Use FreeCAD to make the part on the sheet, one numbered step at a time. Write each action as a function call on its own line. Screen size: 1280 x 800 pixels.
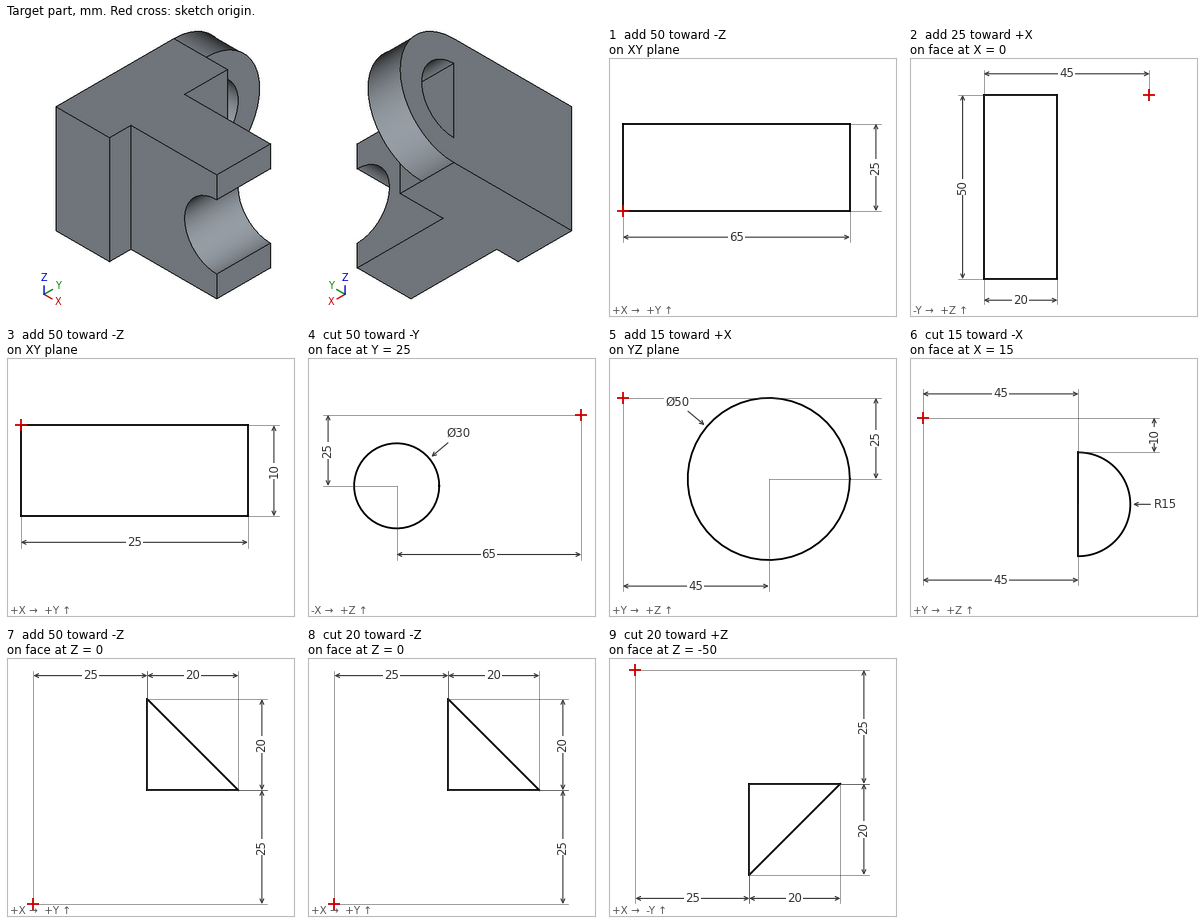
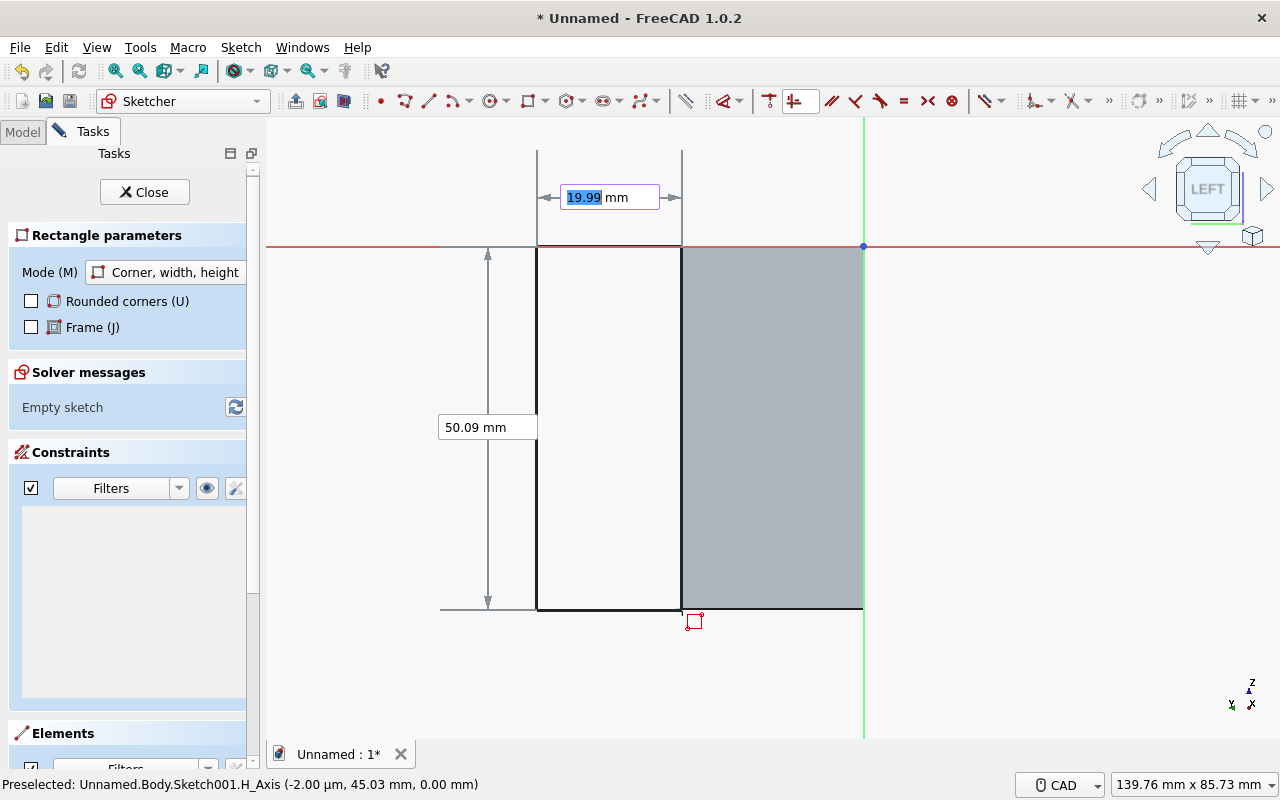
text(20)
key(Tab)
text(50)
key(Return)
key(Escape)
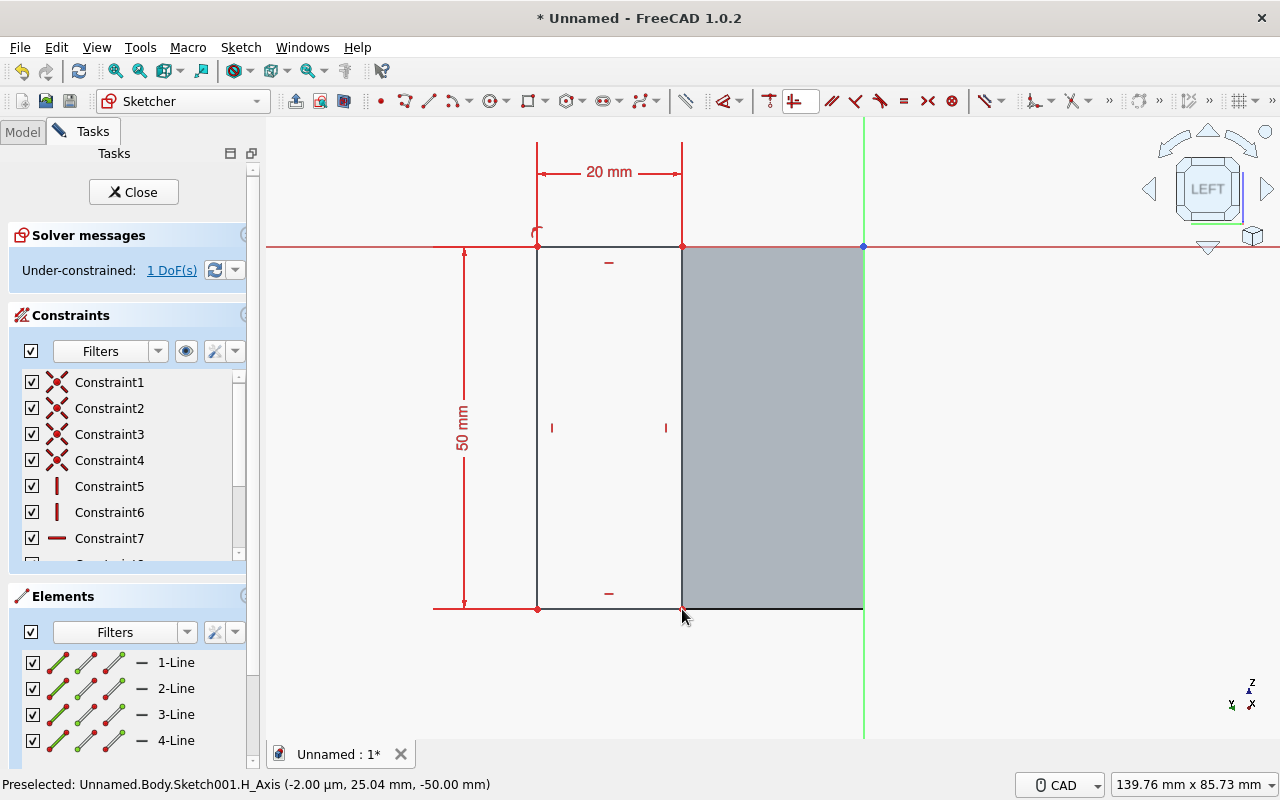
click(537, 247)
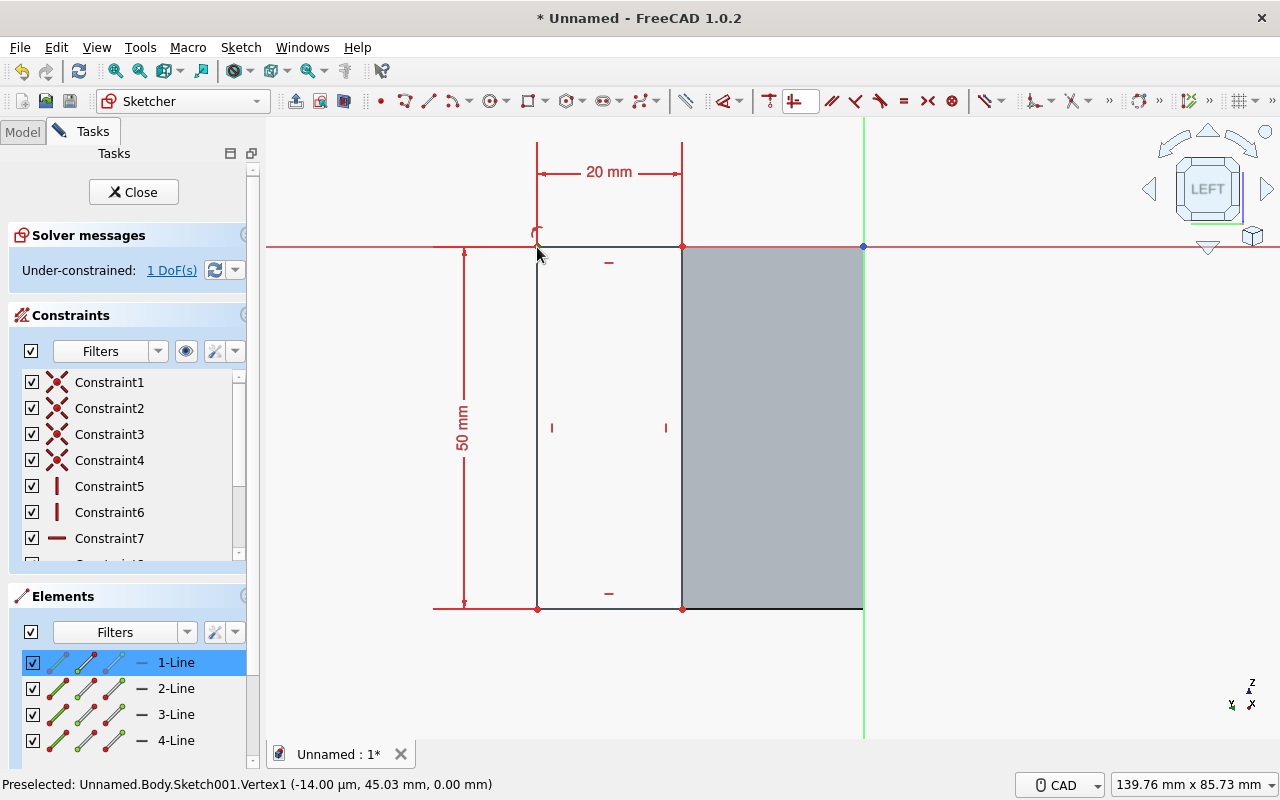
key(l)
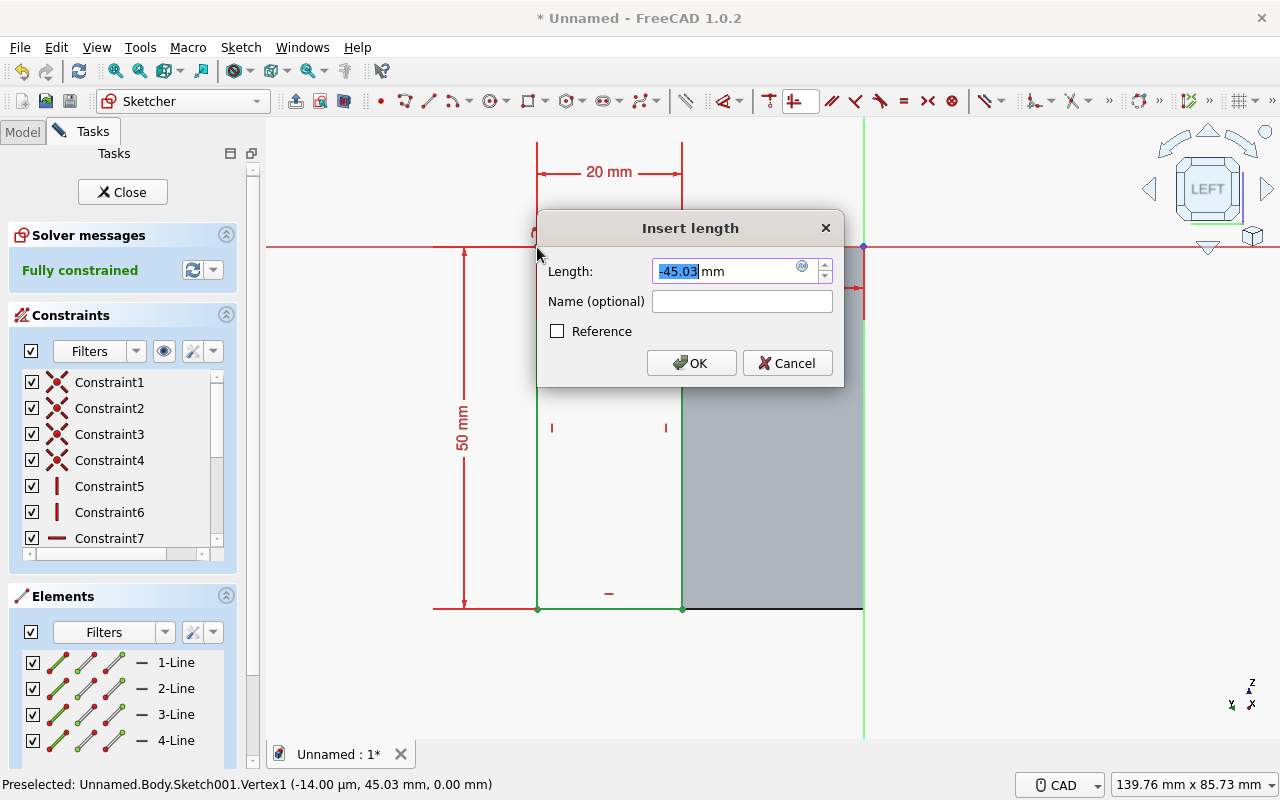
text(-45)
key(Return)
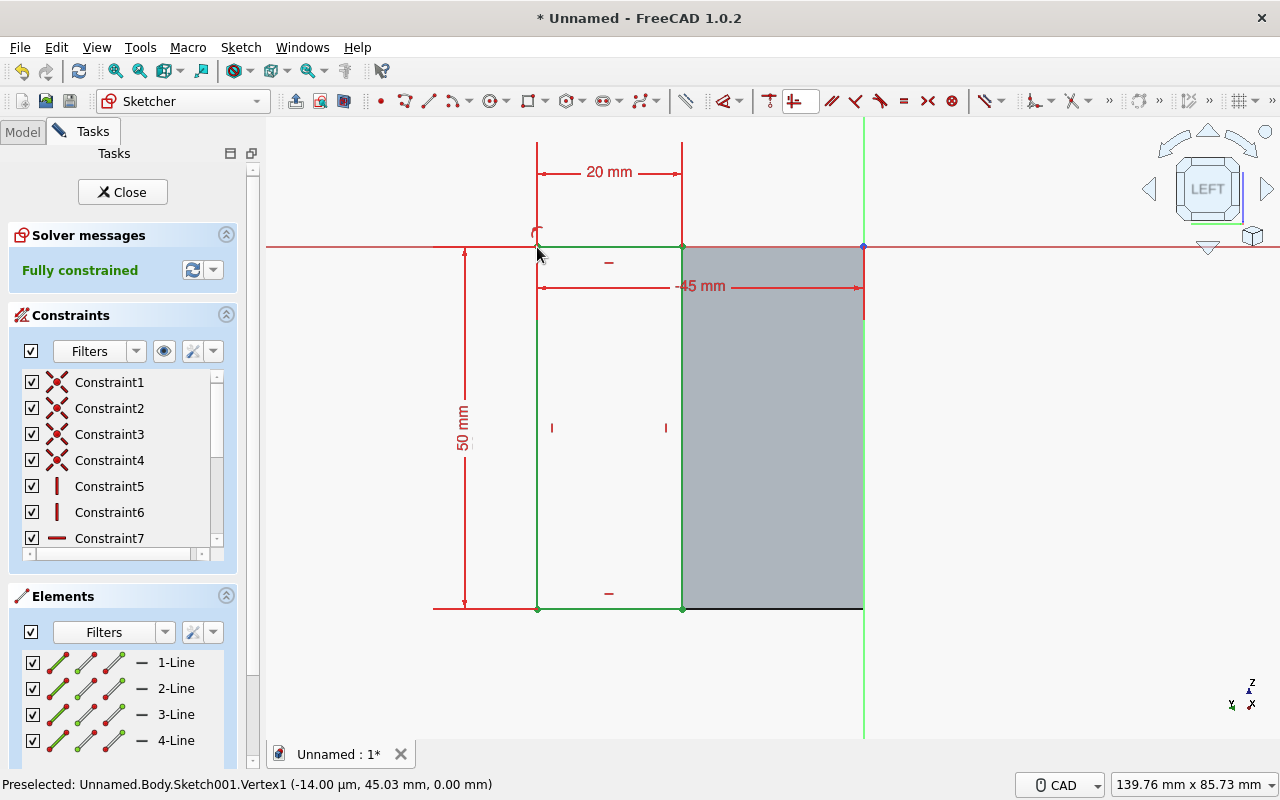
click(123, 192)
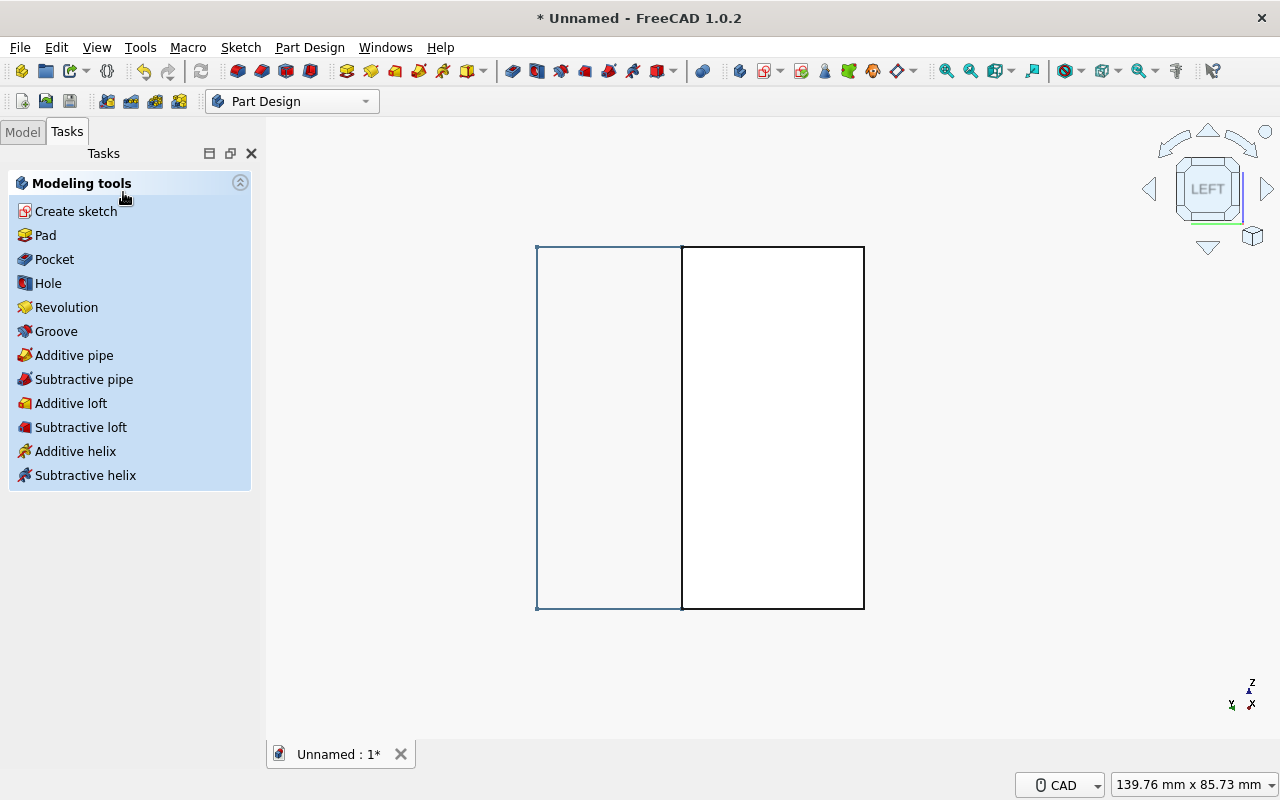
click(348, 72)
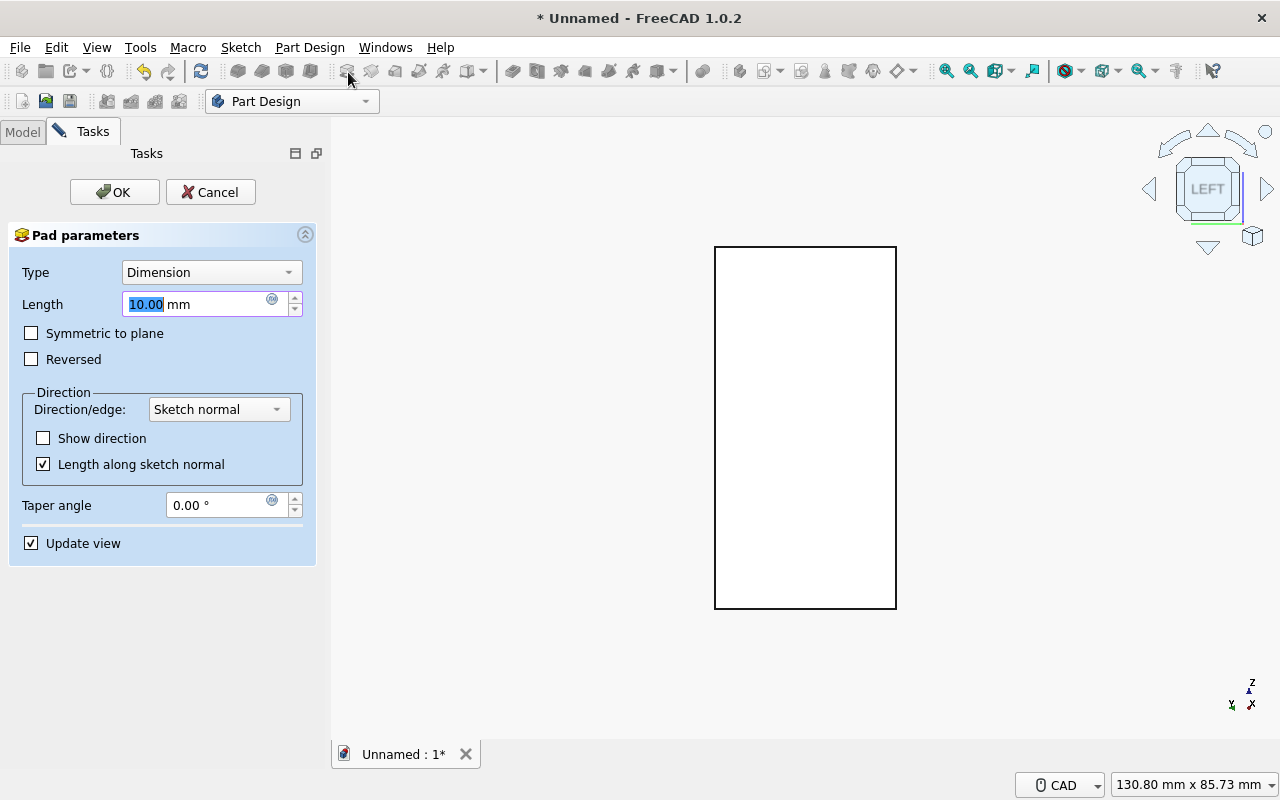
text(25)
key(Tab)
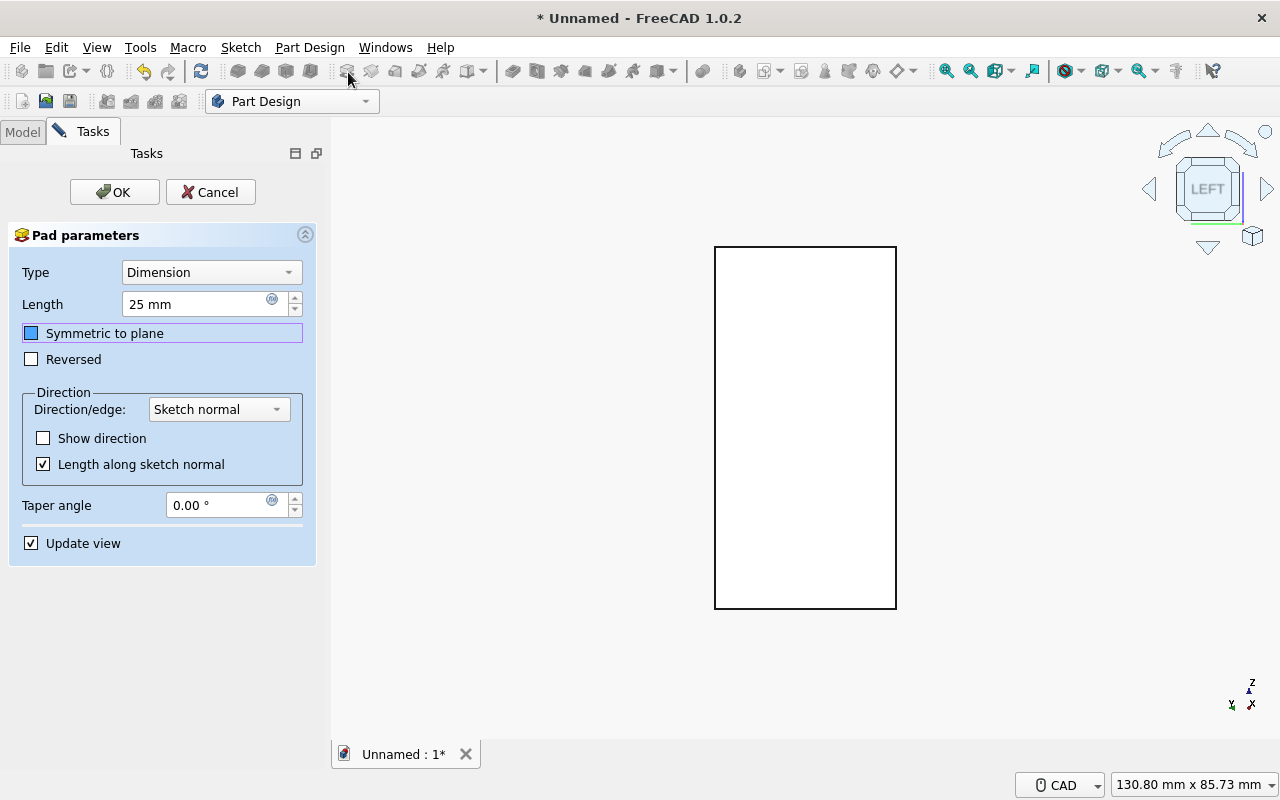
click(30, 359)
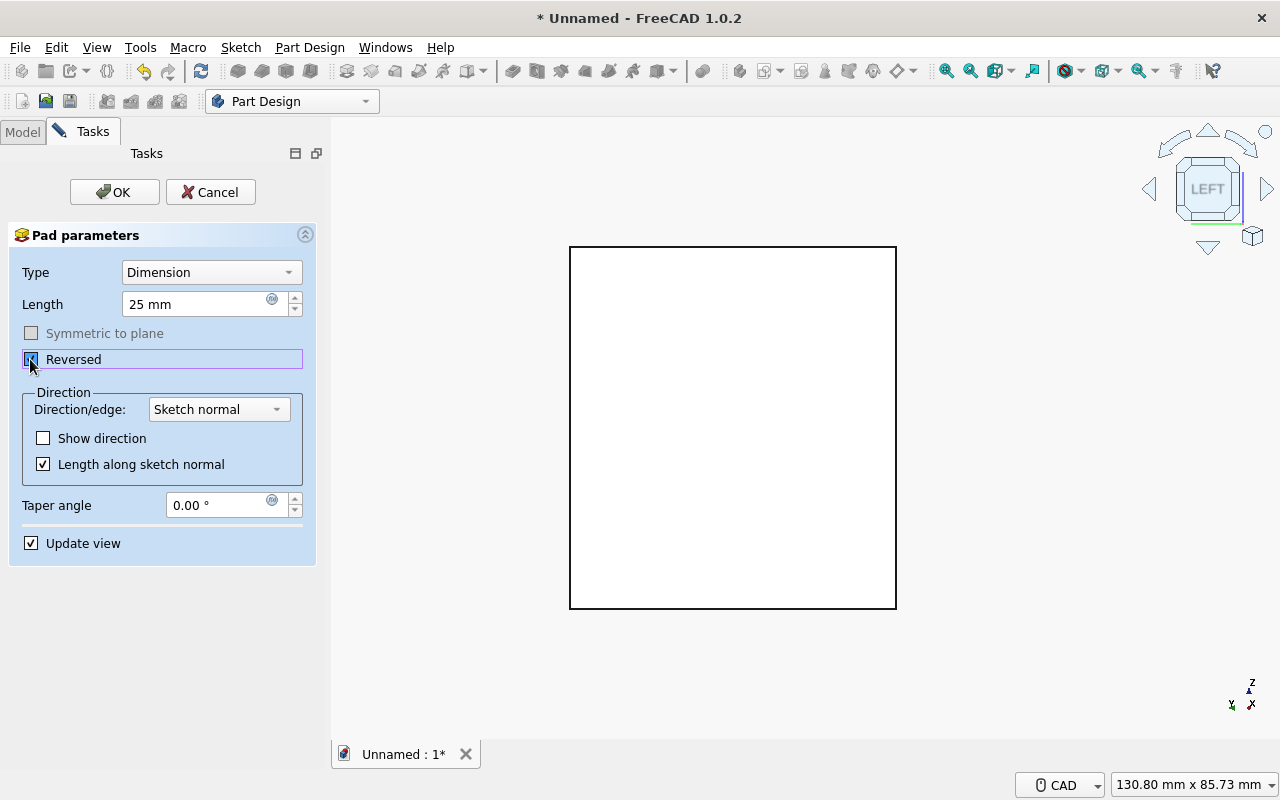
click(115, 192)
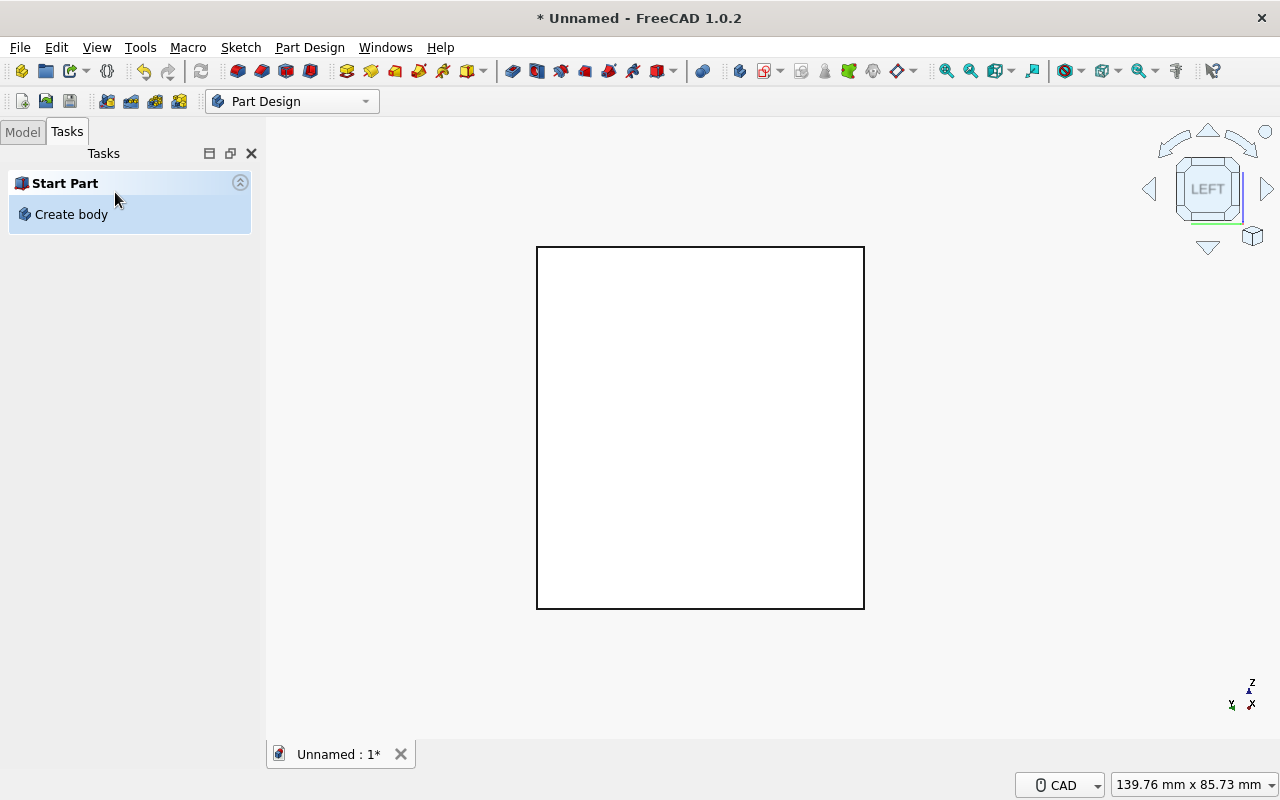
click(764, 72)